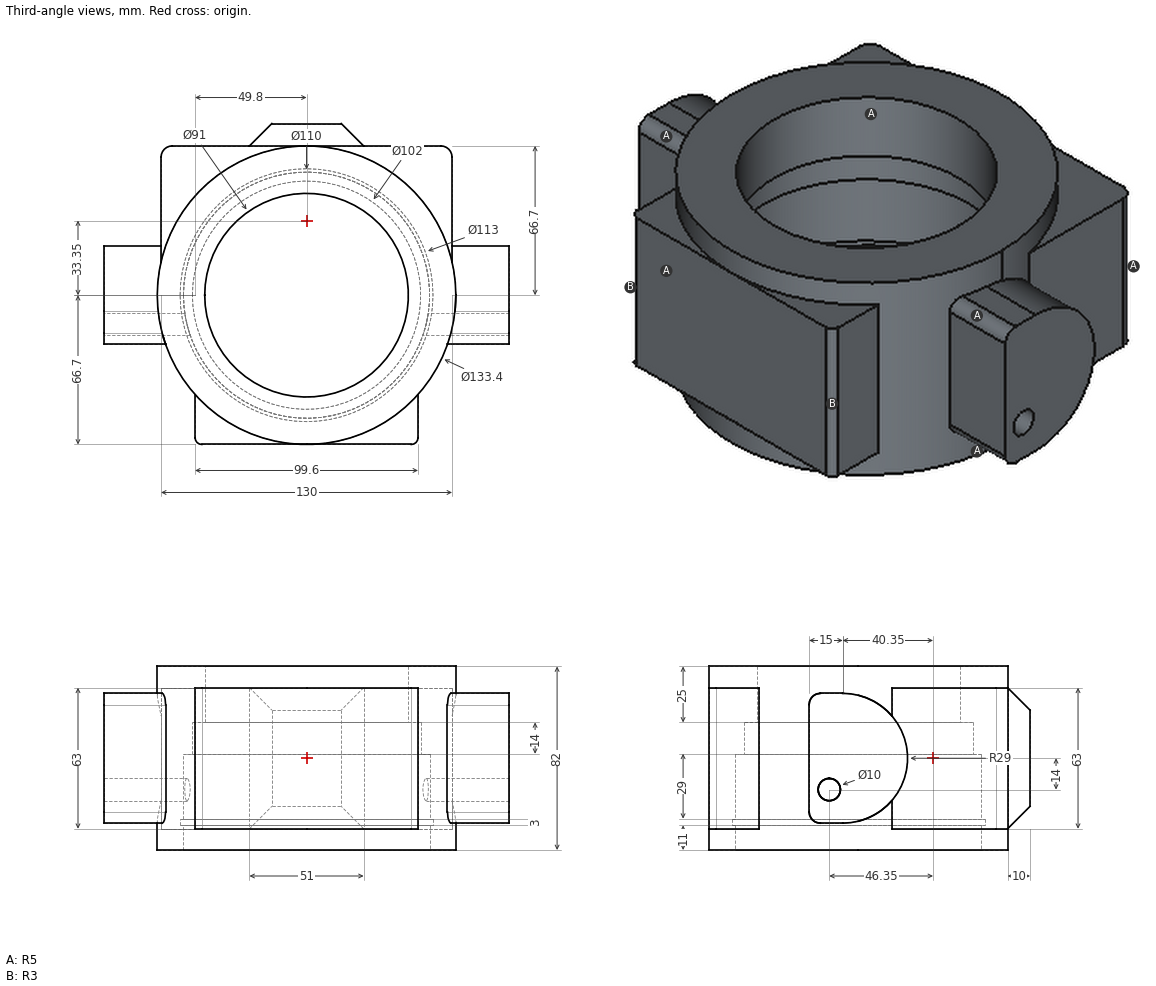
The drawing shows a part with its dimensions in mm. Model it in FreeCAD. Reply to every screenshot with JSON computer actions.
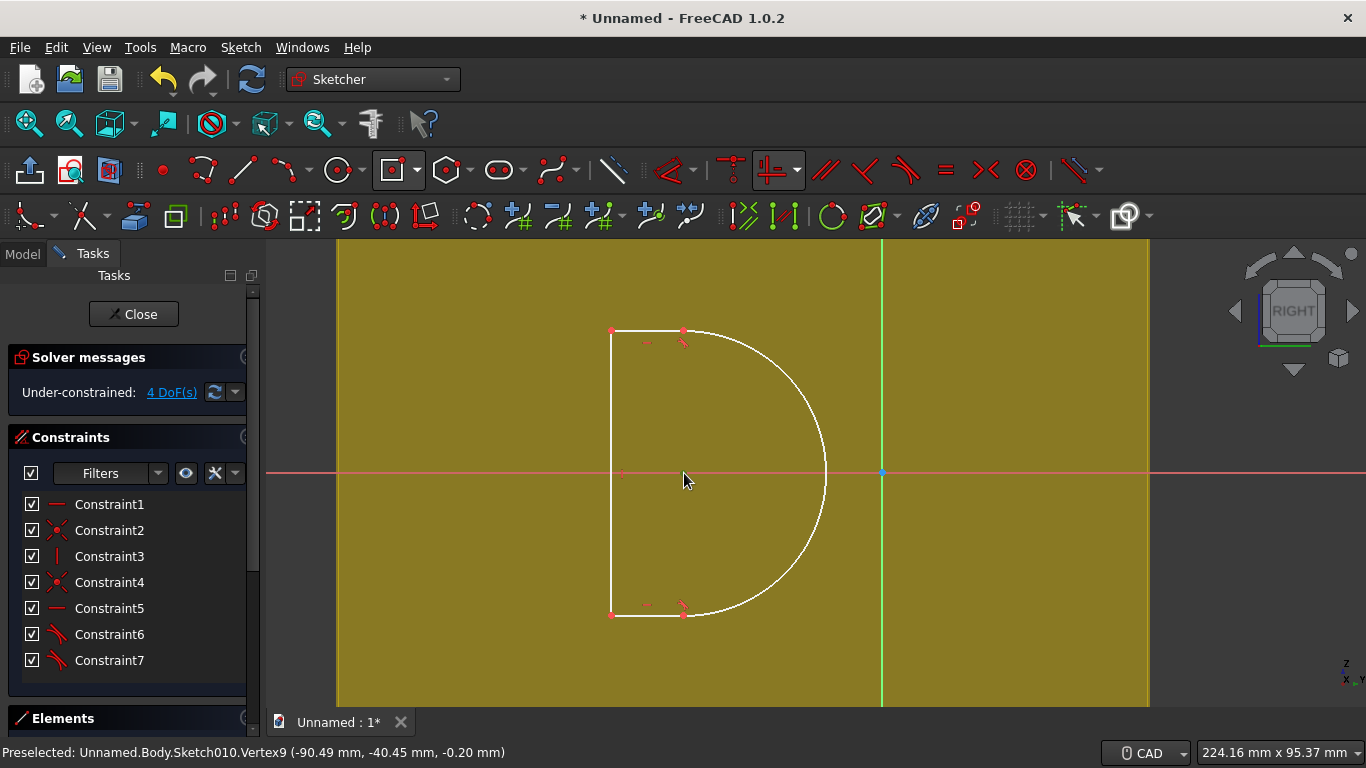
{"action": "left_click", "coordinate": [359, 473]}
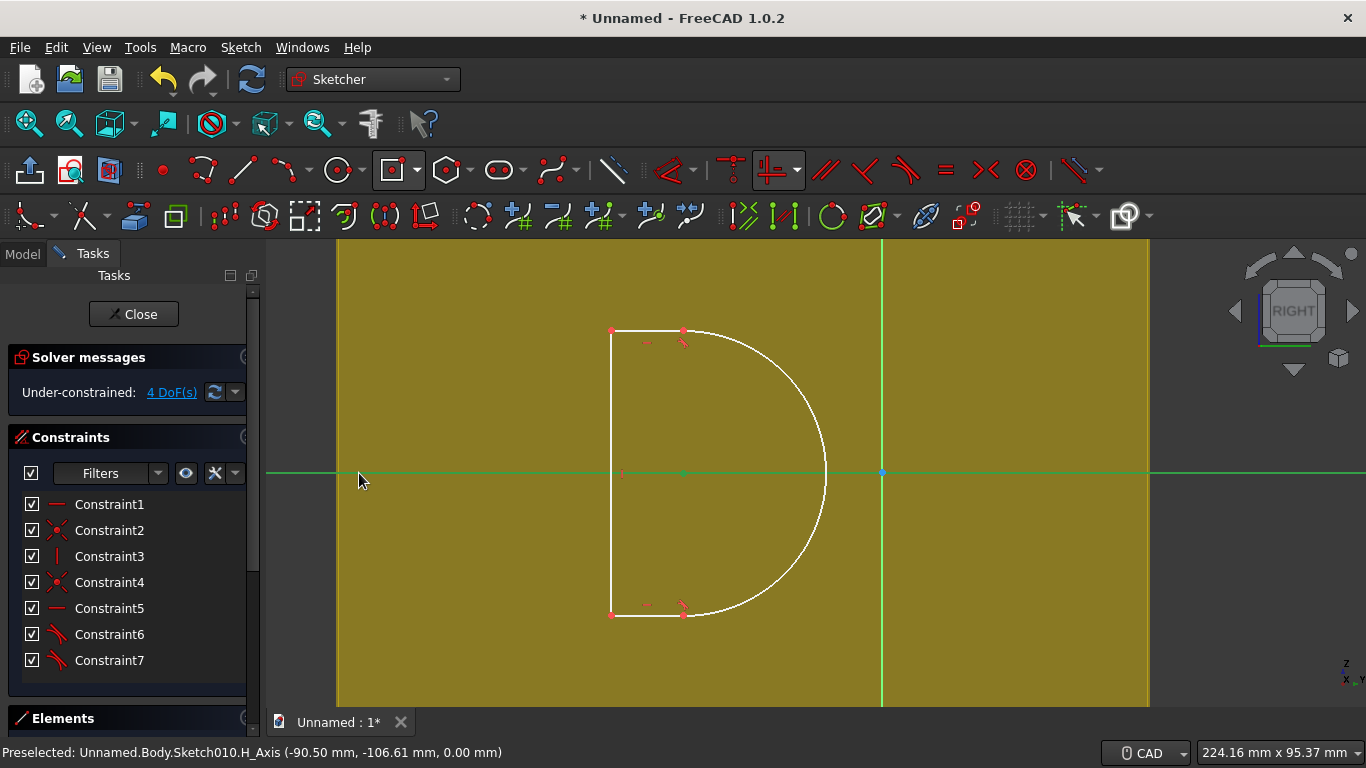
{"action": "left_click", "coordinate": [732, 170]}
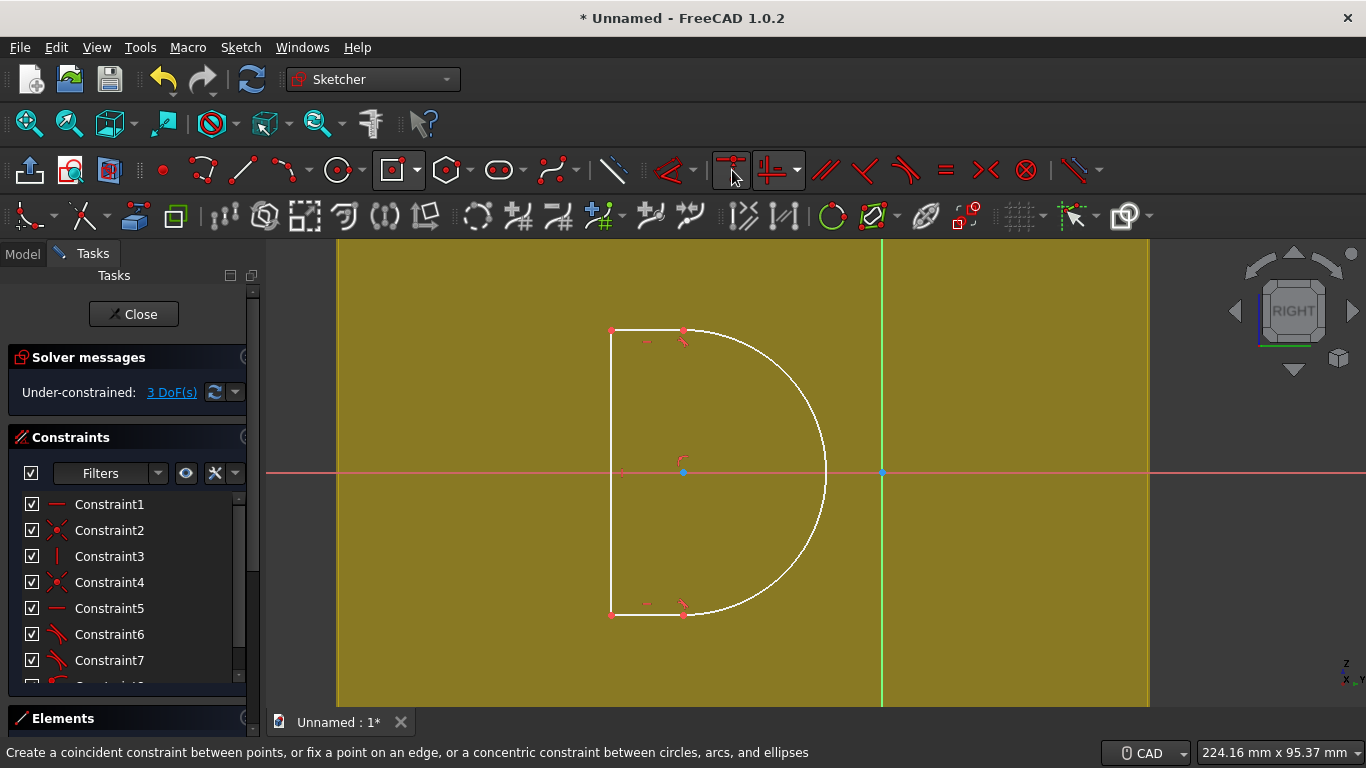
{"action": "key", "text": "d"}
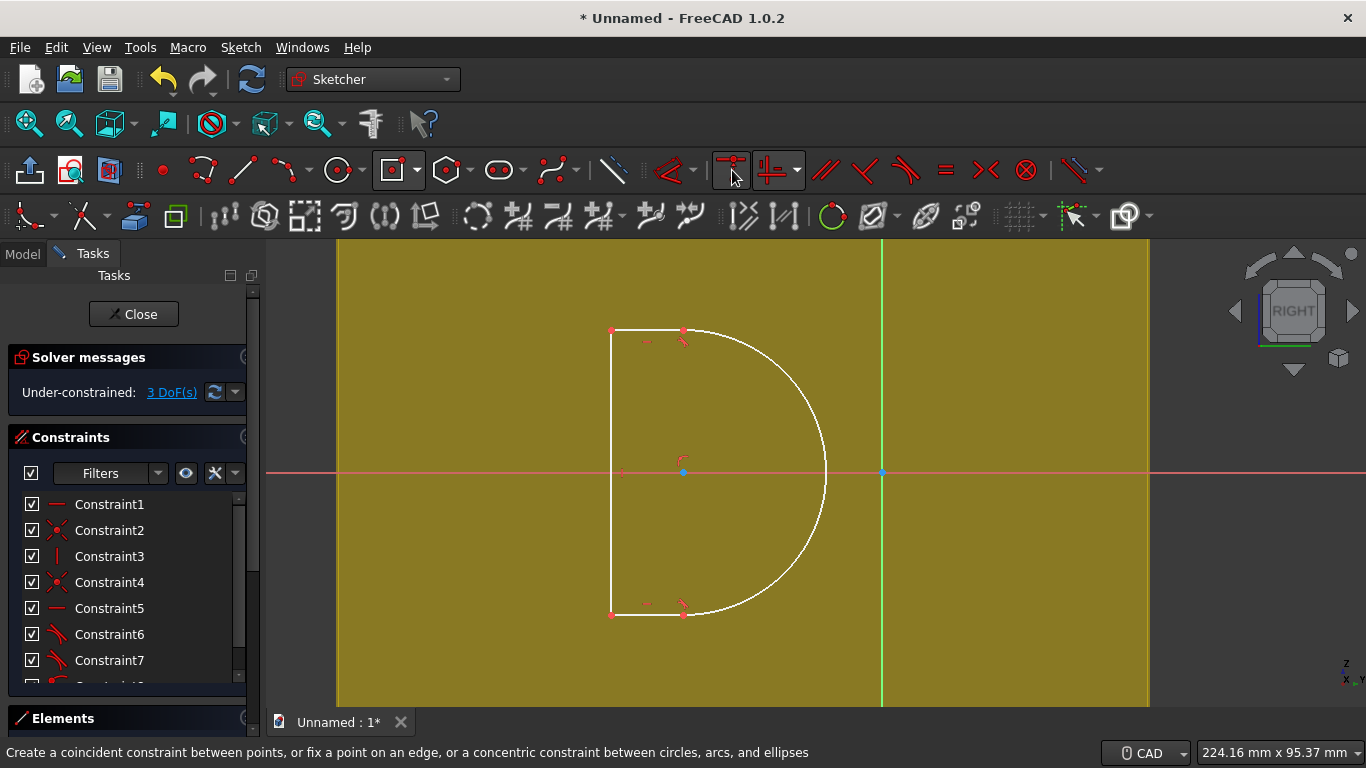
{"action": "left_click", "coordinate": [799, 556]}
{"action": "left_click", "coordinate": [825, 575]}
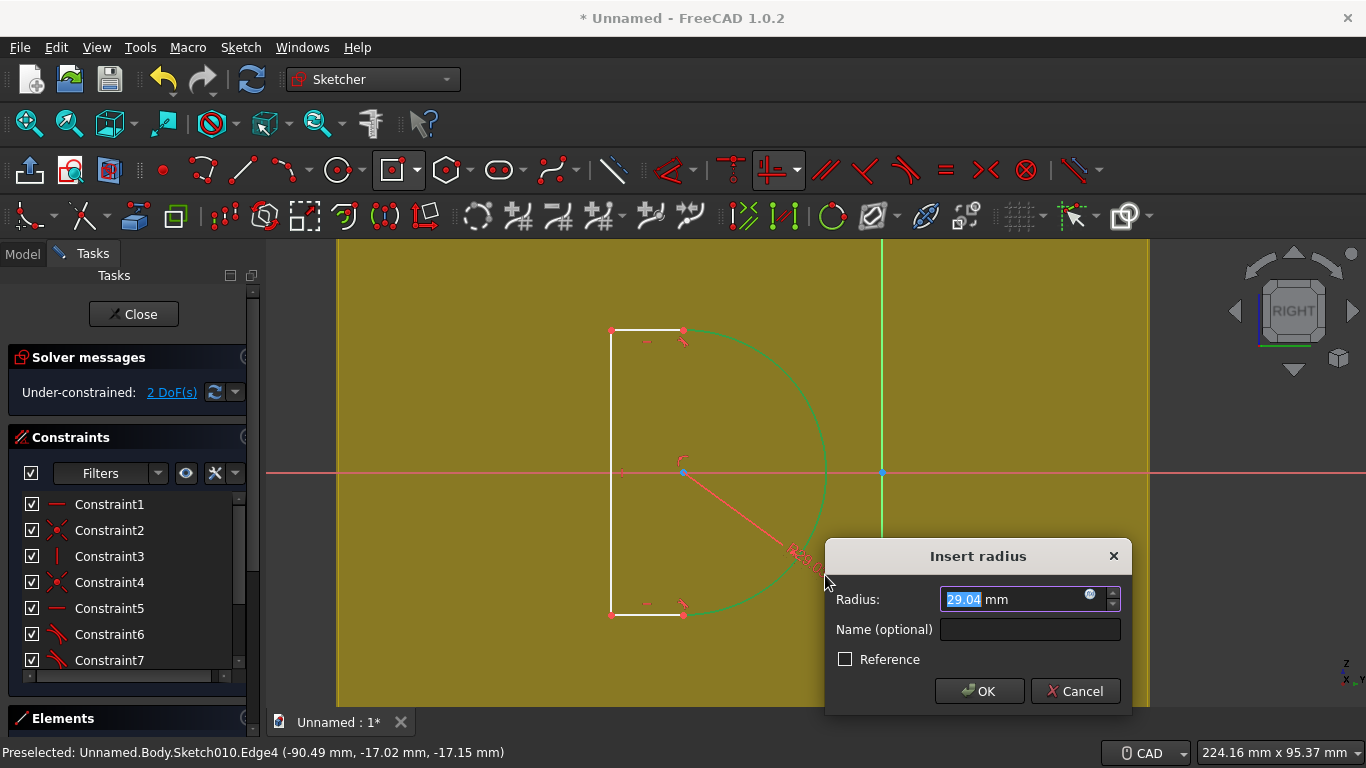
{"action": "type", "text": "29"}
{"action": "key", "text": "Return"}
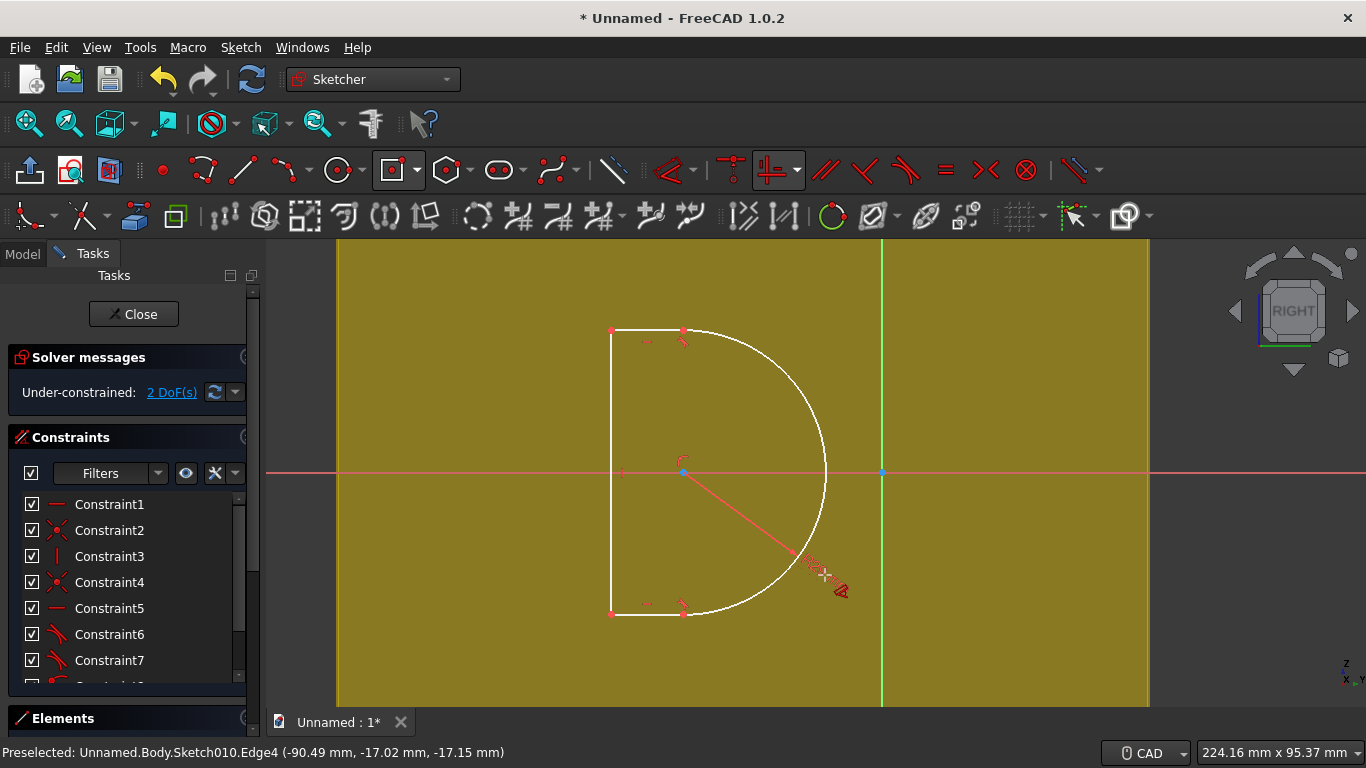
{"action": "left_click", "coordinate": [662, 330]}
{"action": "left_click", "coordinate": [647, 296]}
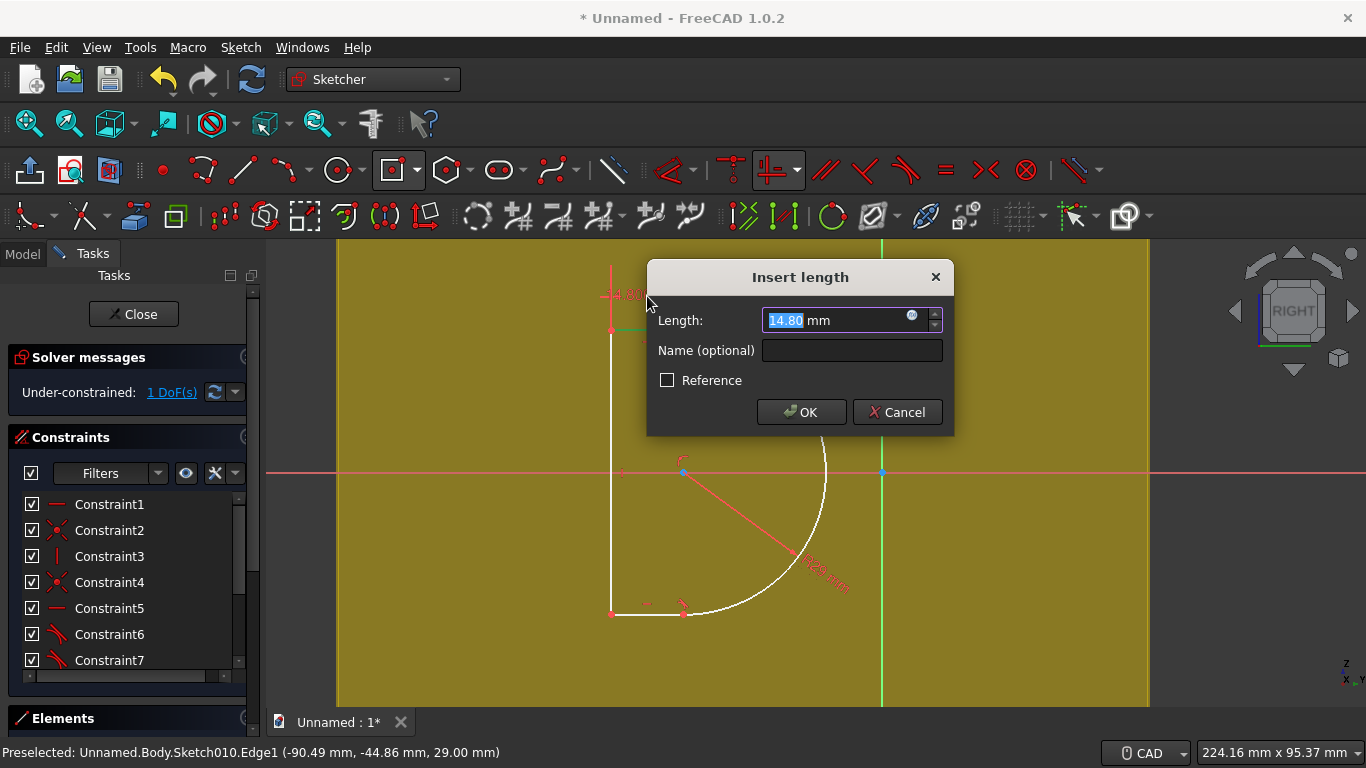
{"action": "type", "text": "15"}
{"action": "key", "text": "Return"}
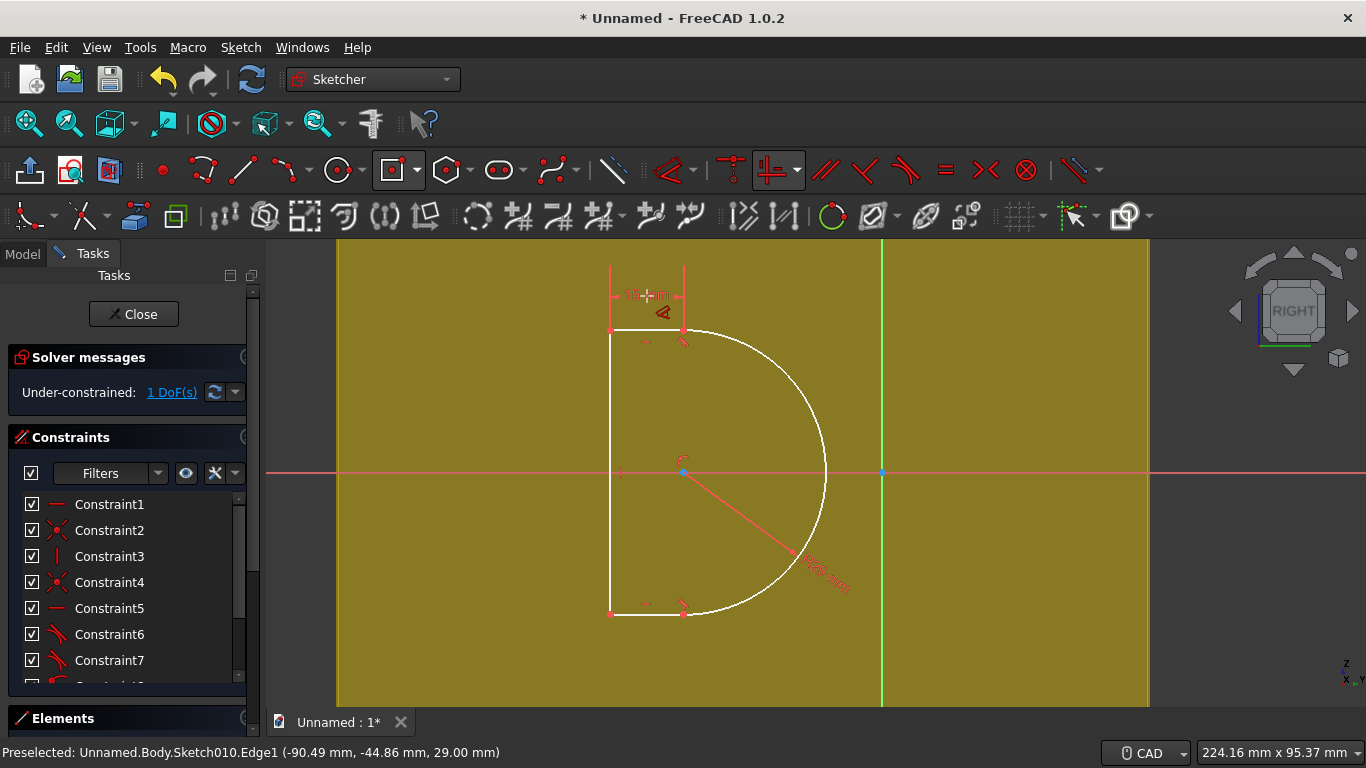
{"action": "left_click", "coordinate": [684, 330]}
{"action": "left_click", "coordinate": [783, 296]}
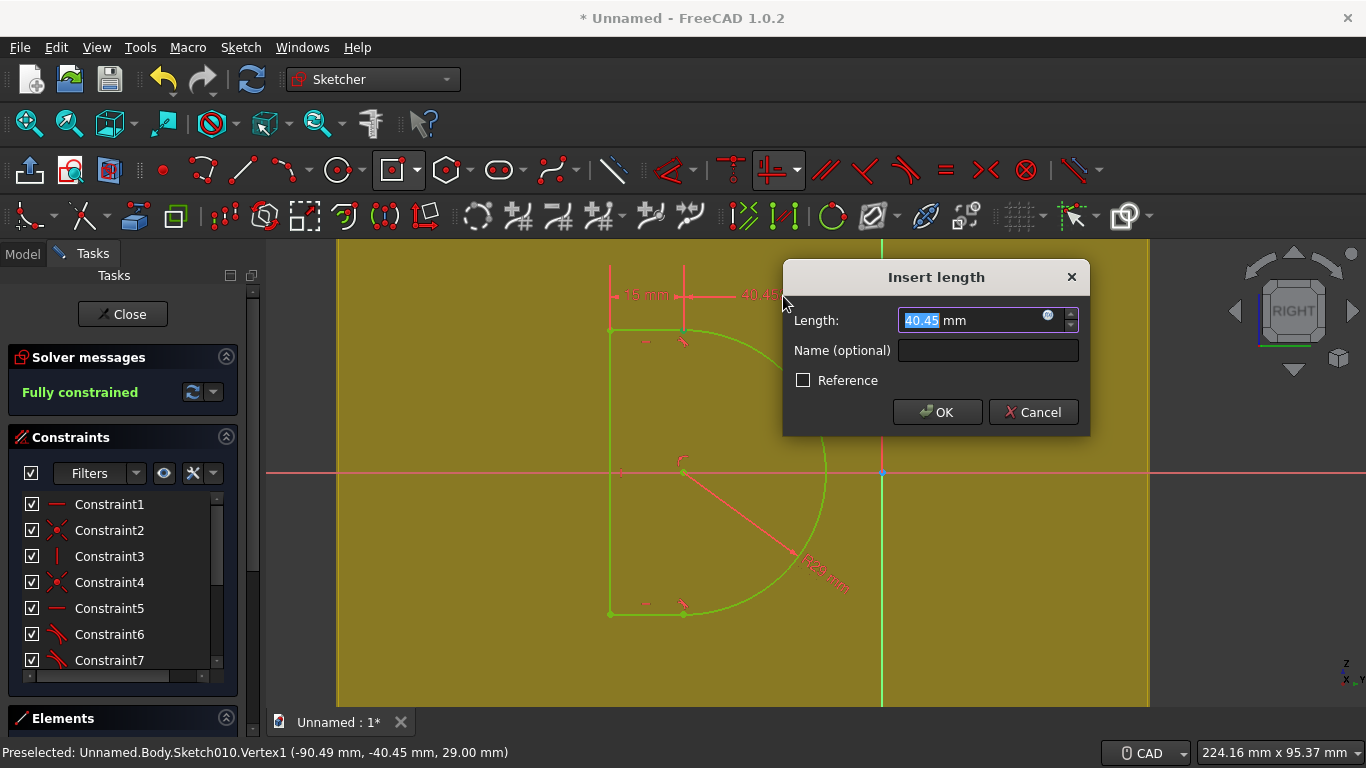
{"action": "type", "text": "40.35"}
{"action": "key", "text": "Return"}
{"action": "key", "text": "Escape"}